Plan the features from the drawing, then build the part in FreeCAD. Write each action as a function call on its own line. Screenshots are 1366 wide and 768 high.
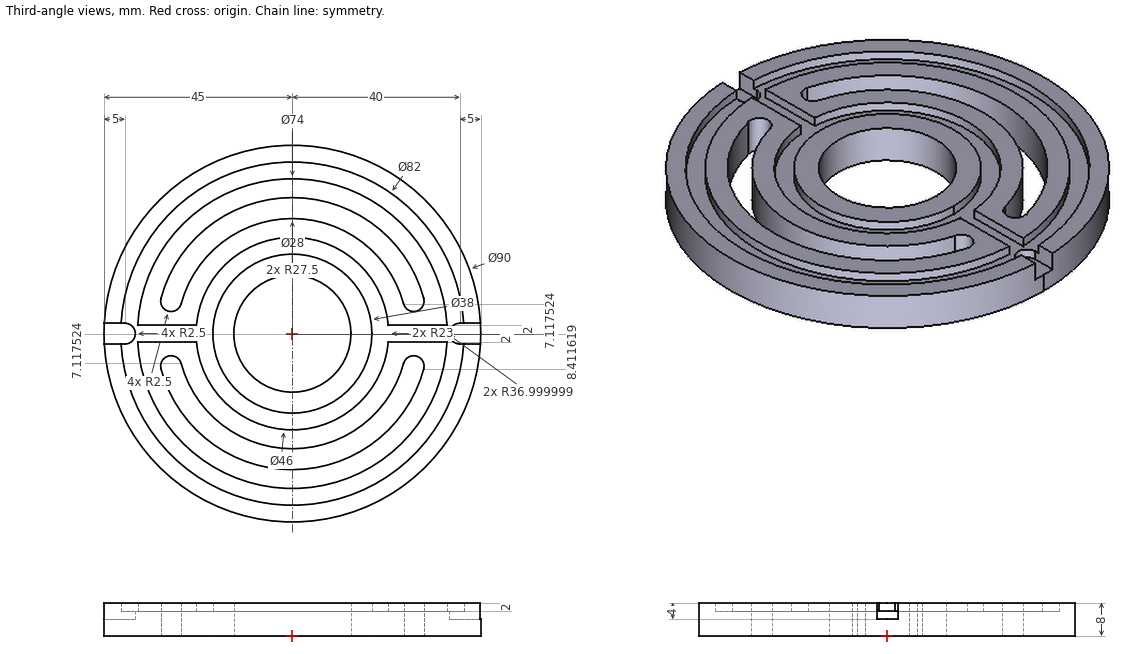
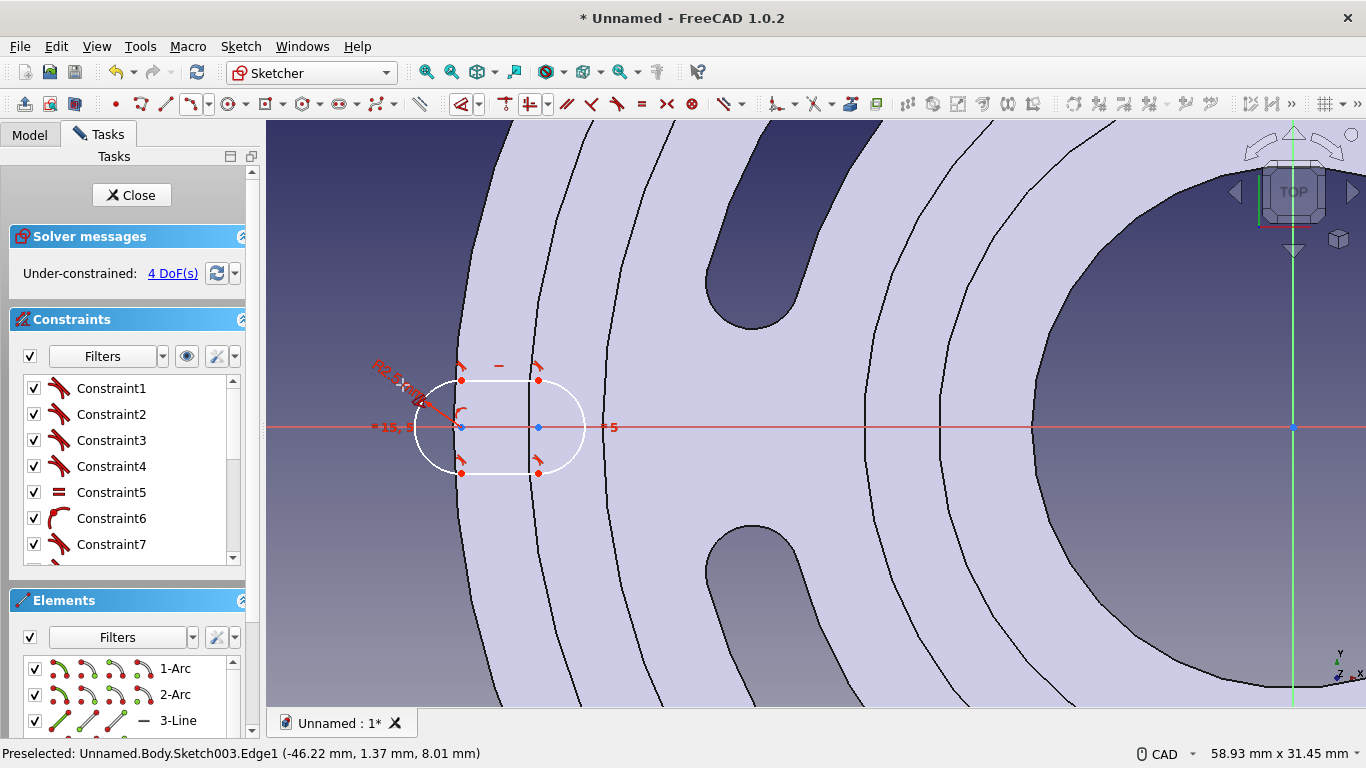
click(484, 381)
click(500, 347)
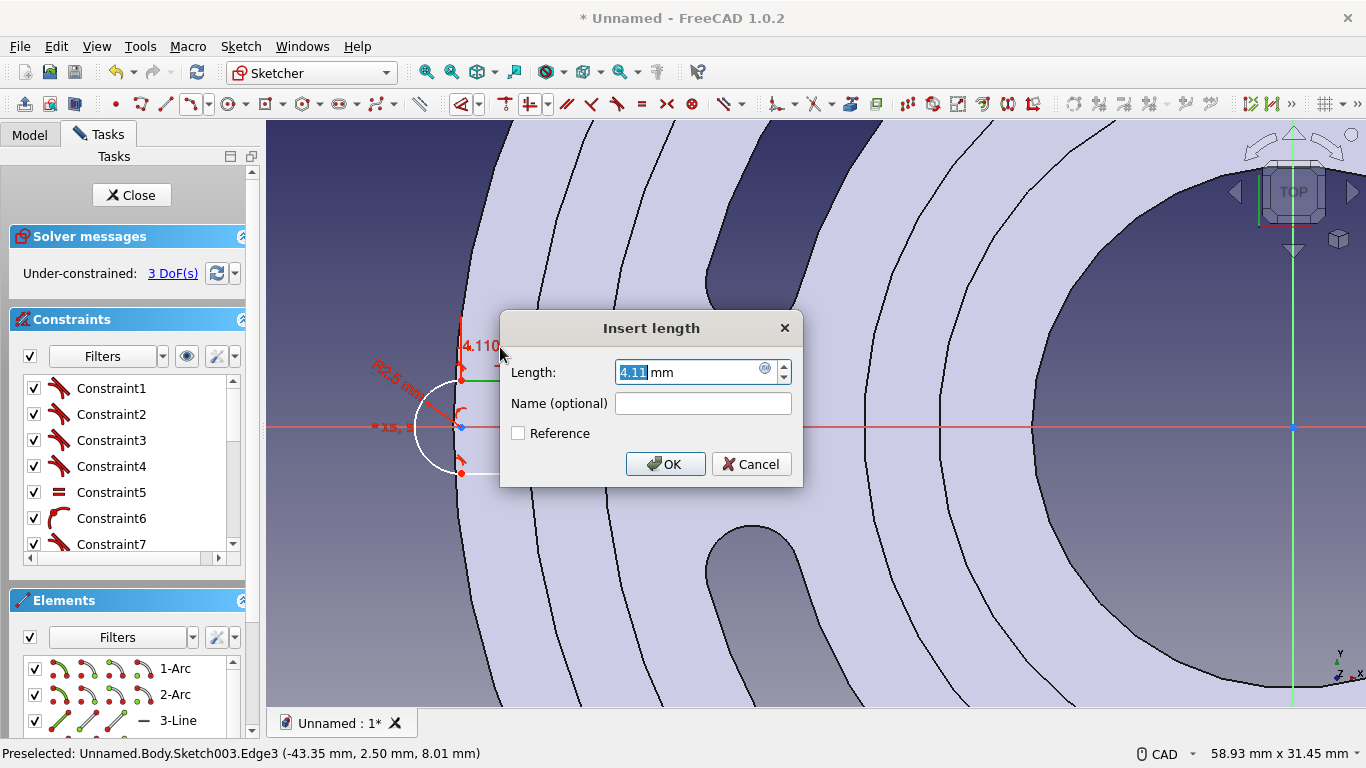
text(5)
key(Return)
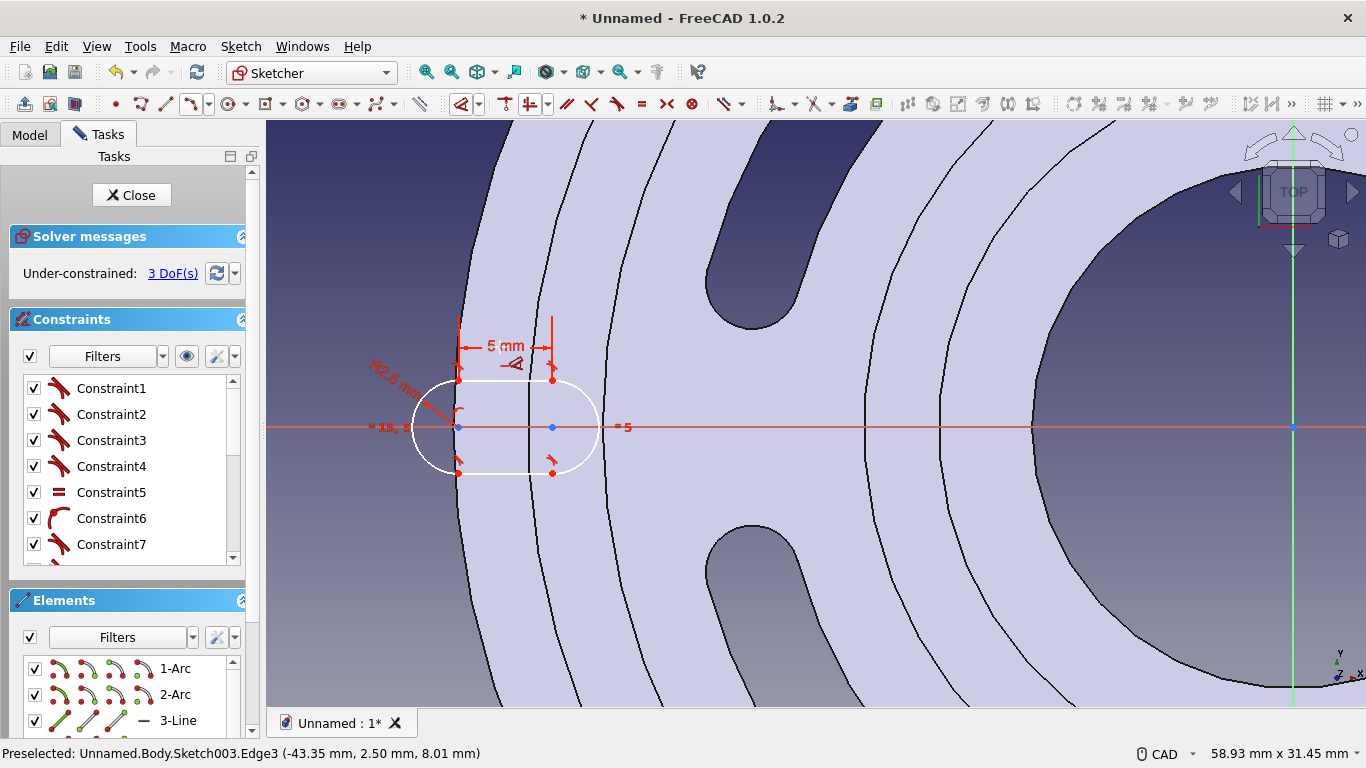
scroll(430, 405, down, 5)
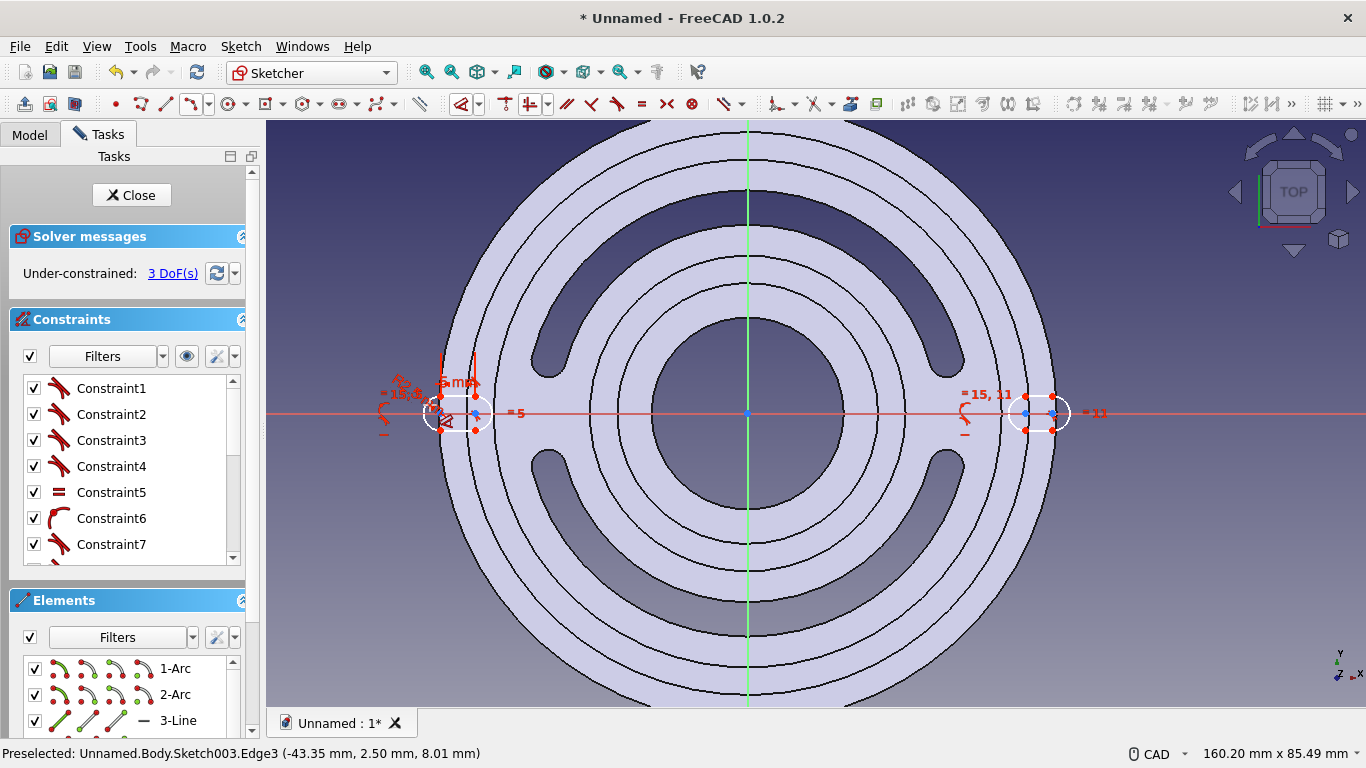
scroll(1034, 396, up, 3)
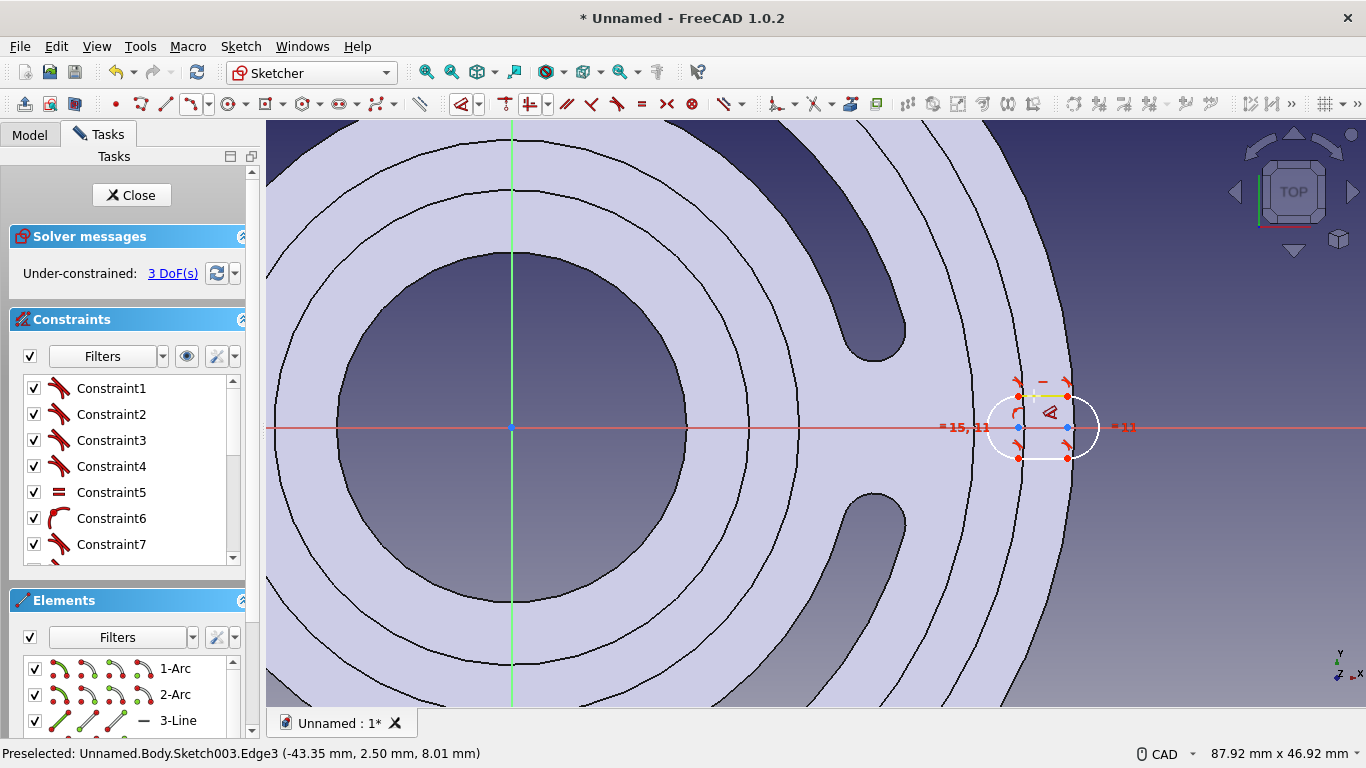
click(1033, 396)
click(1043, 362)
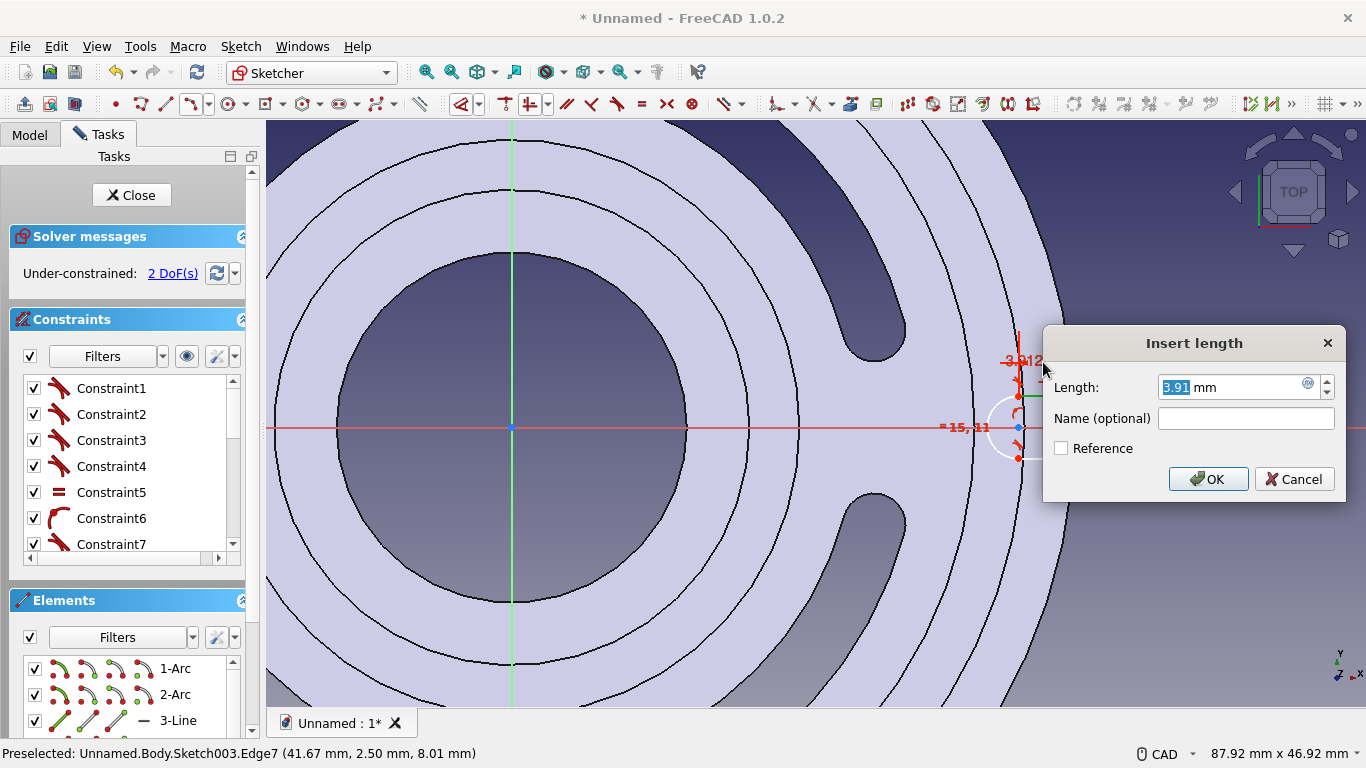
text(5)
key(Return)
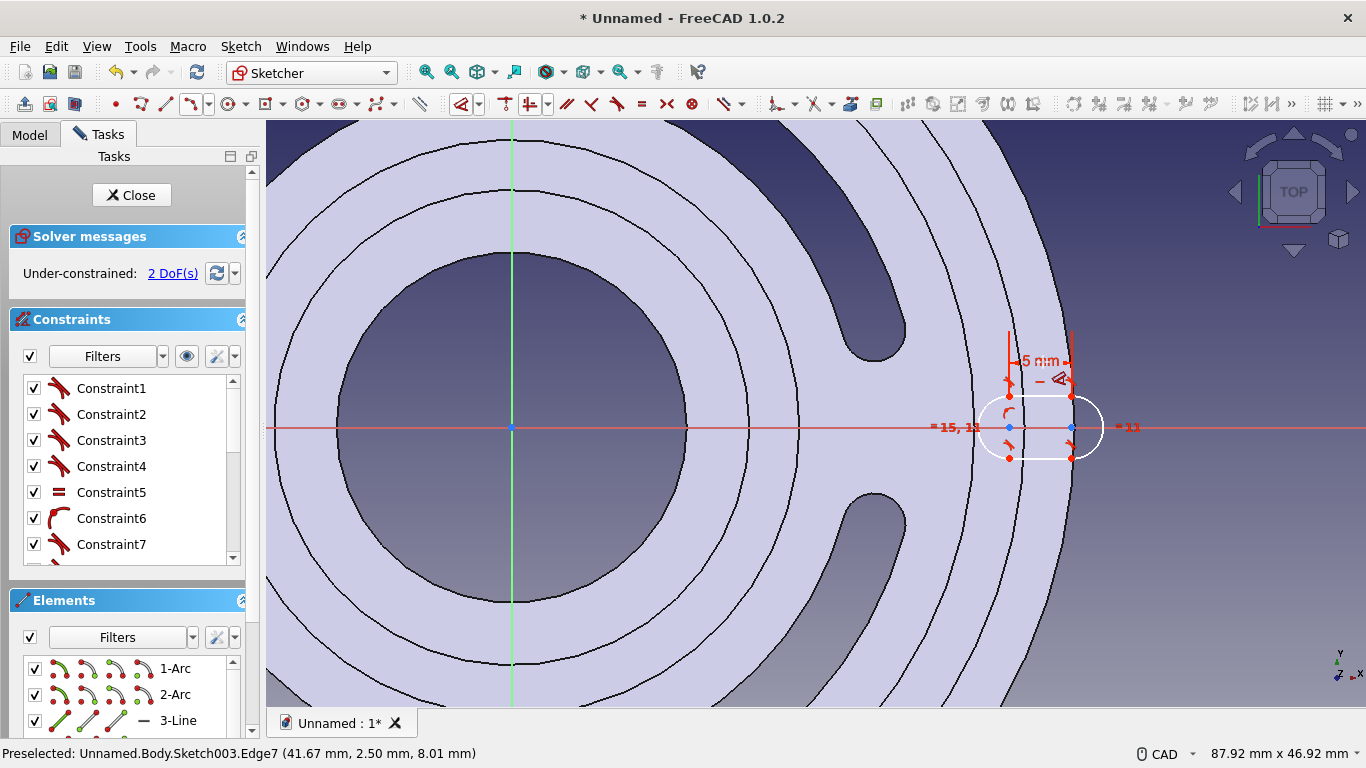
scroll(1034, 396, down, 3)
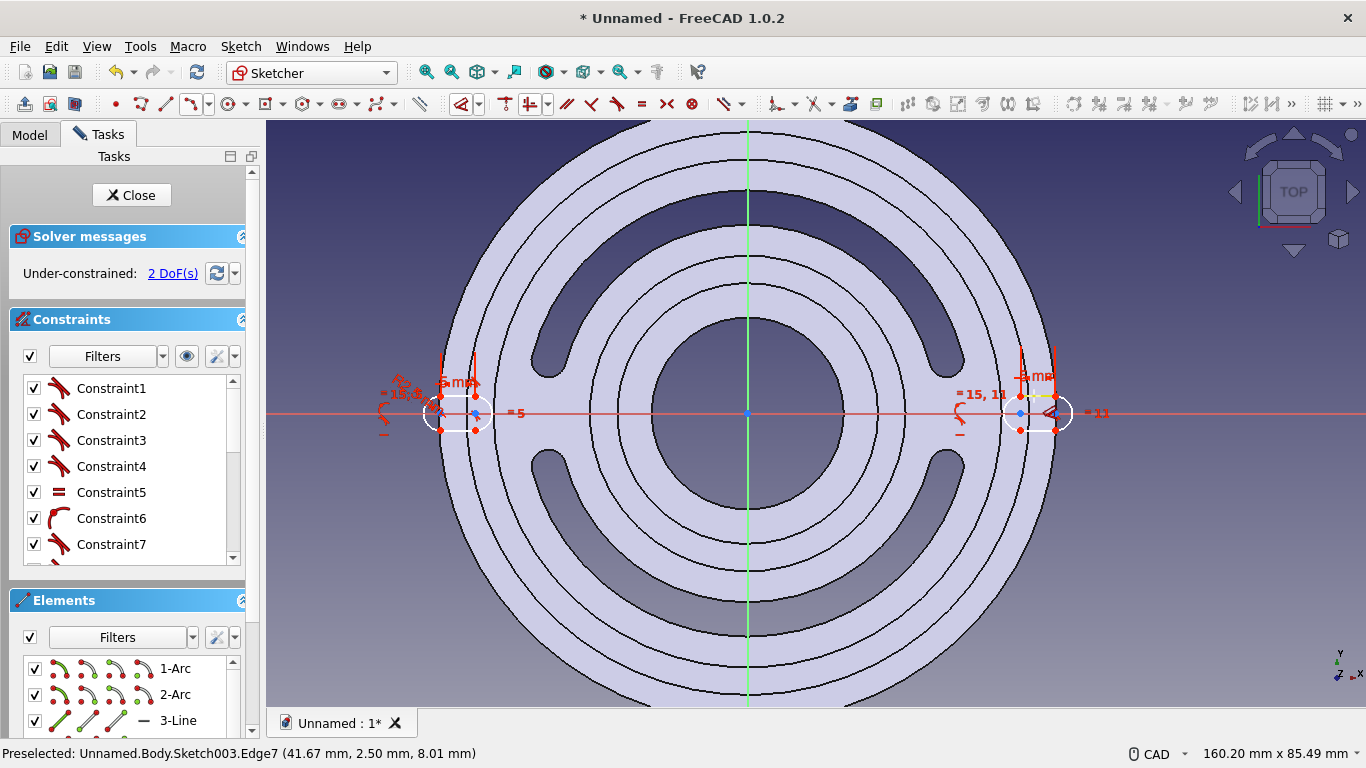
click(441, 396)
click(594, 362)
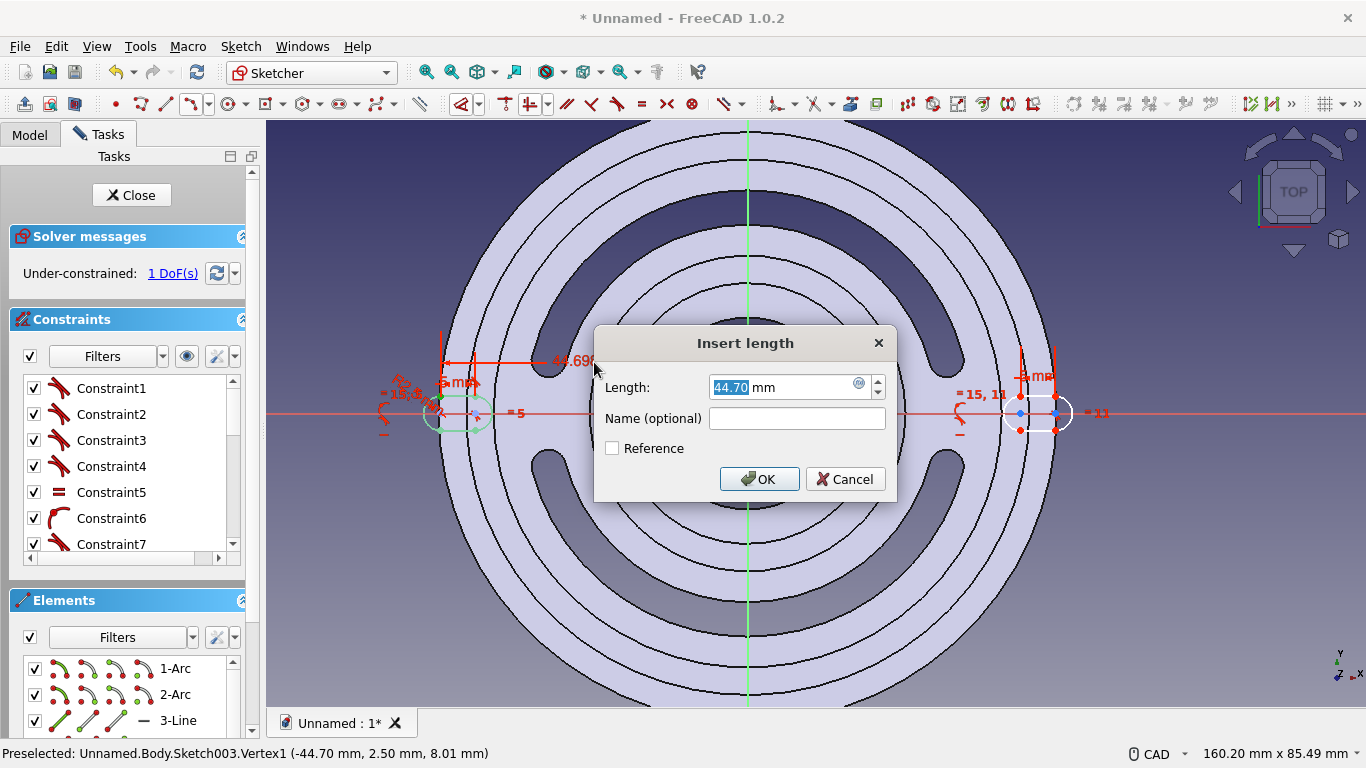
text(45)
key(Return)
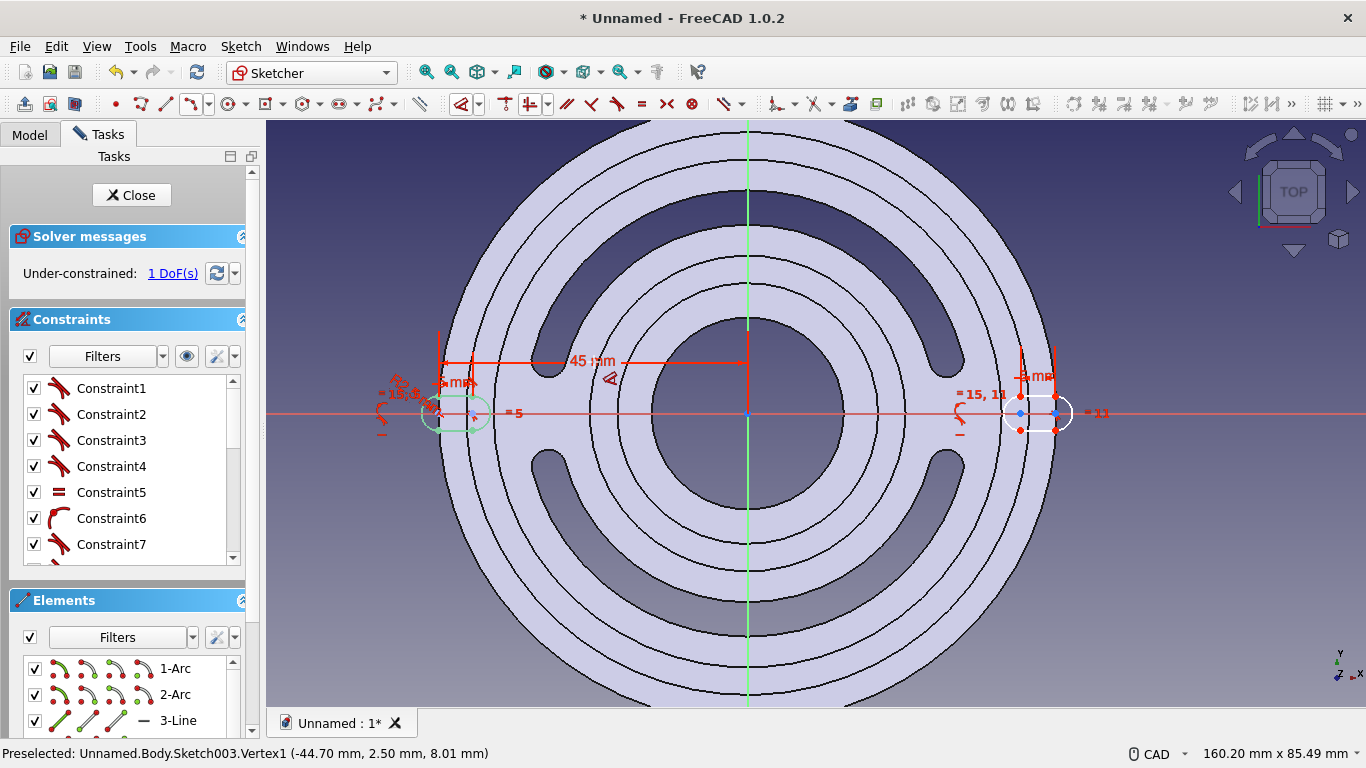
click(1021, 396)
click(884, 362)